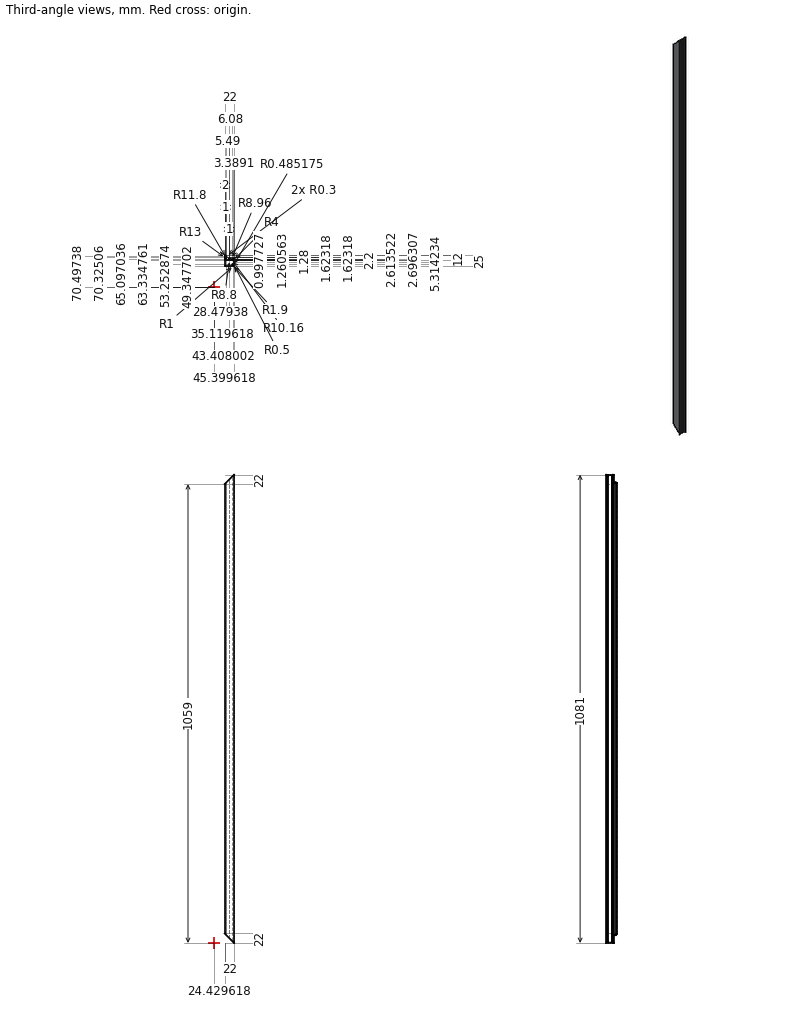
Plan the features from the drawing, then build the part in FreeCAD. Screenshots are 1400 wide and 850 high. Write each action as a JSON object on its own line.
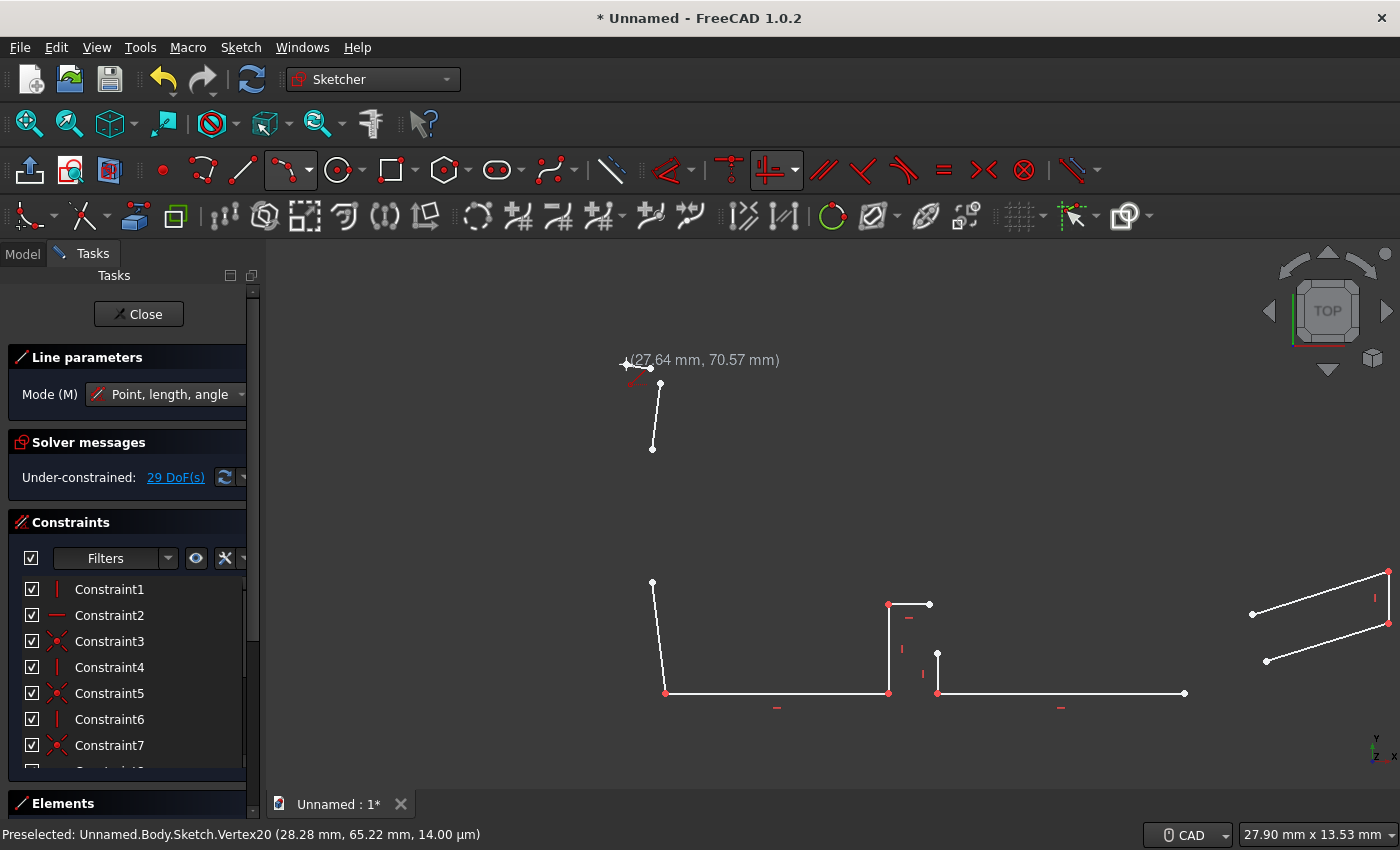
{"action": "left_click", "coordinate": [612, 375]}
{"action": "left_click", "coordinate": [603, 441]}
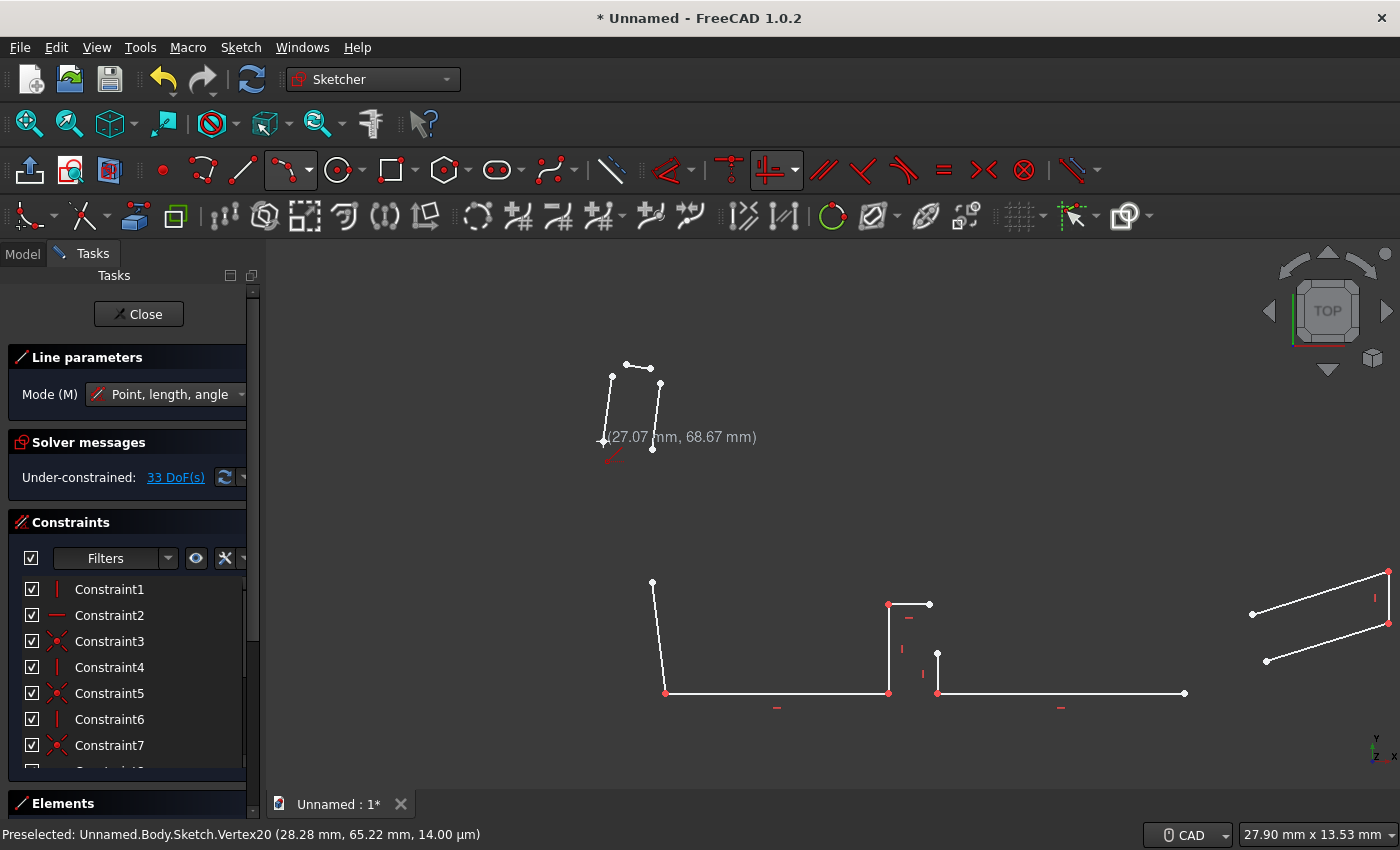
{"action": "left_click", "coordinate": [204, 170]}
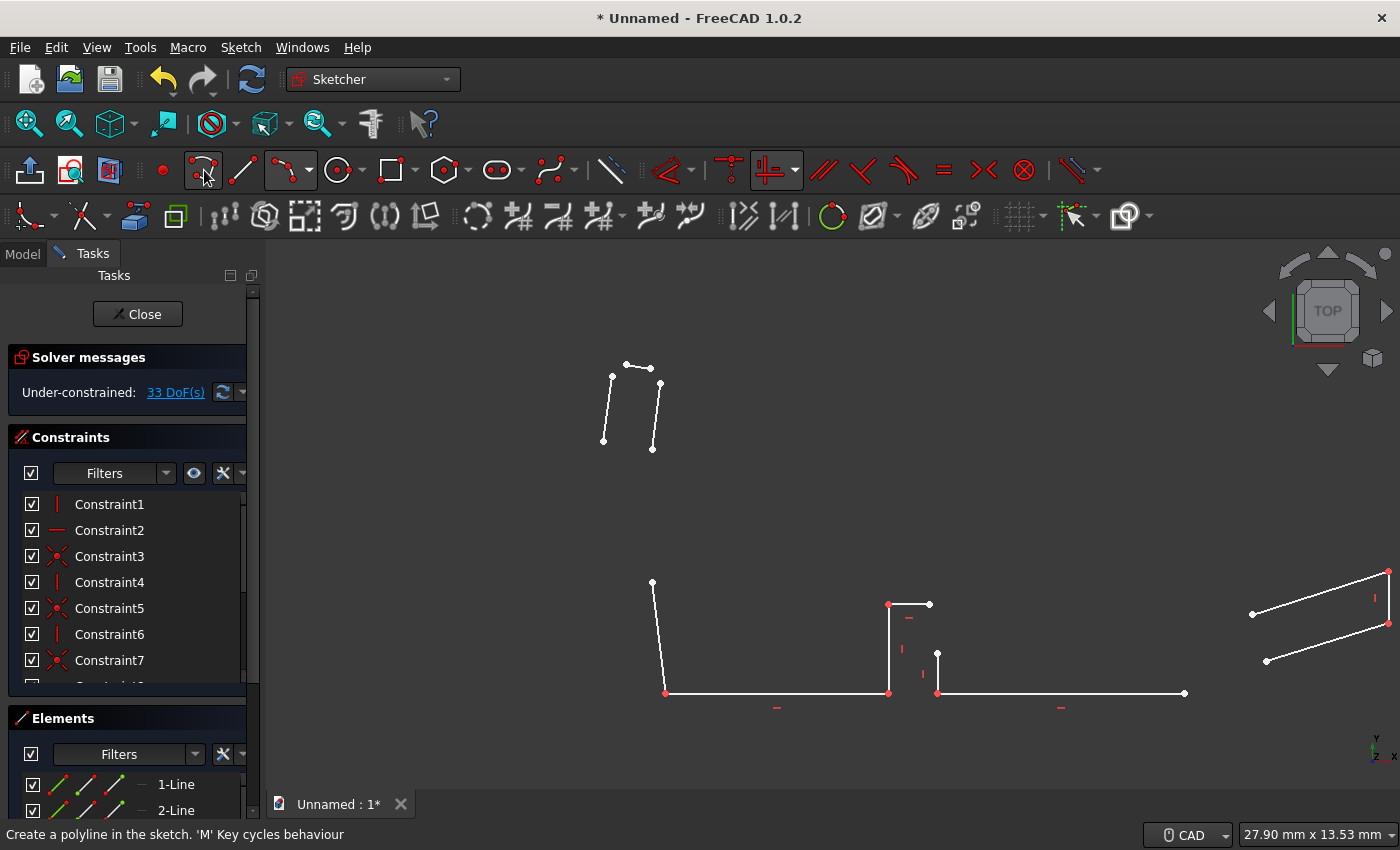
{"action": "left_click", "coordinate": [603, 587]}
{"action": "left_click", "coordinate": [618, 693]}
{"action": "left_click", "coordinate": [618, 745]}
{"action": "left_click", "coordinate": [577, 745]}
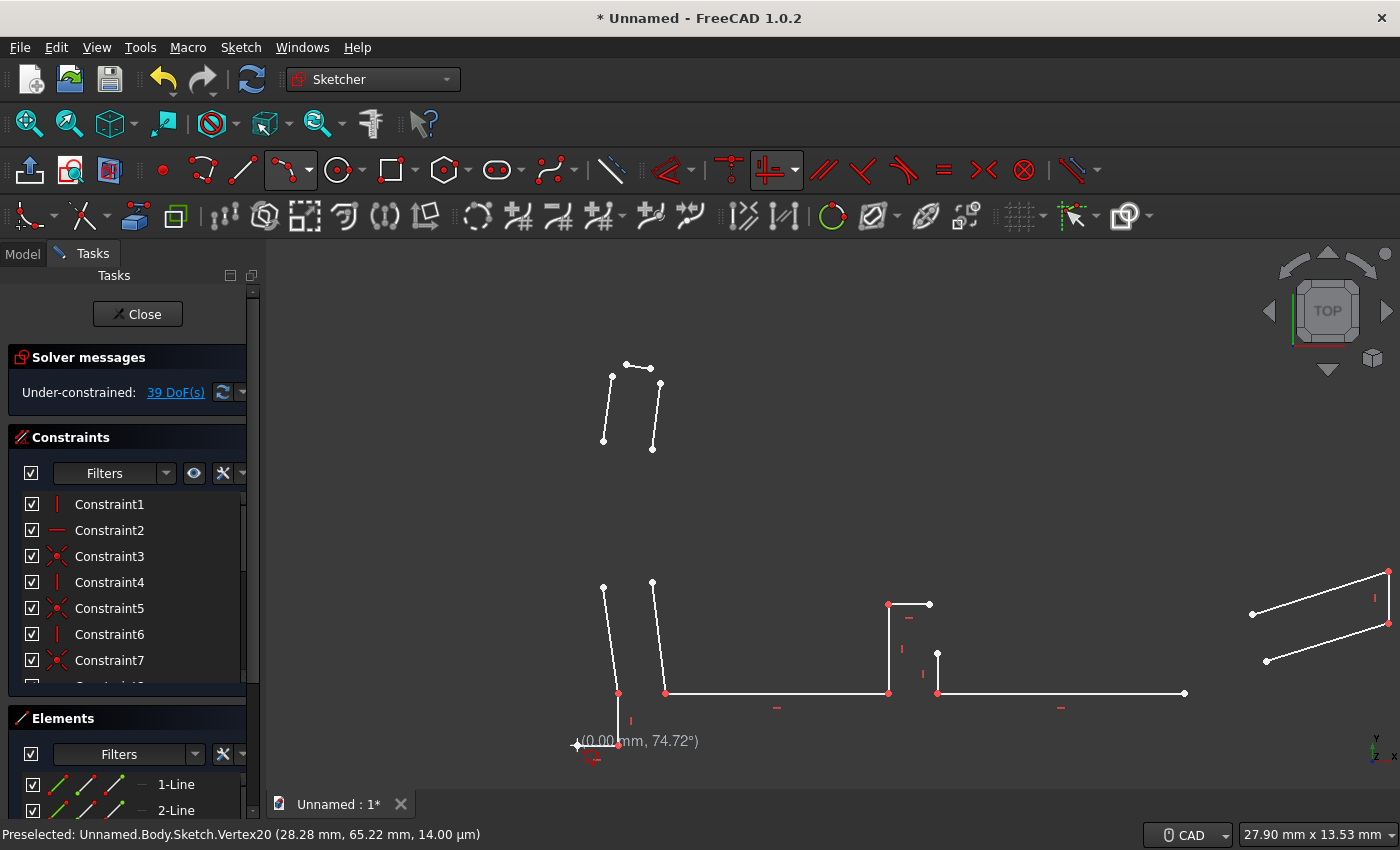
{"action": "scroll", "coordinate": [661, 367], "scroll_direction": "down", "scroll_amount": 5}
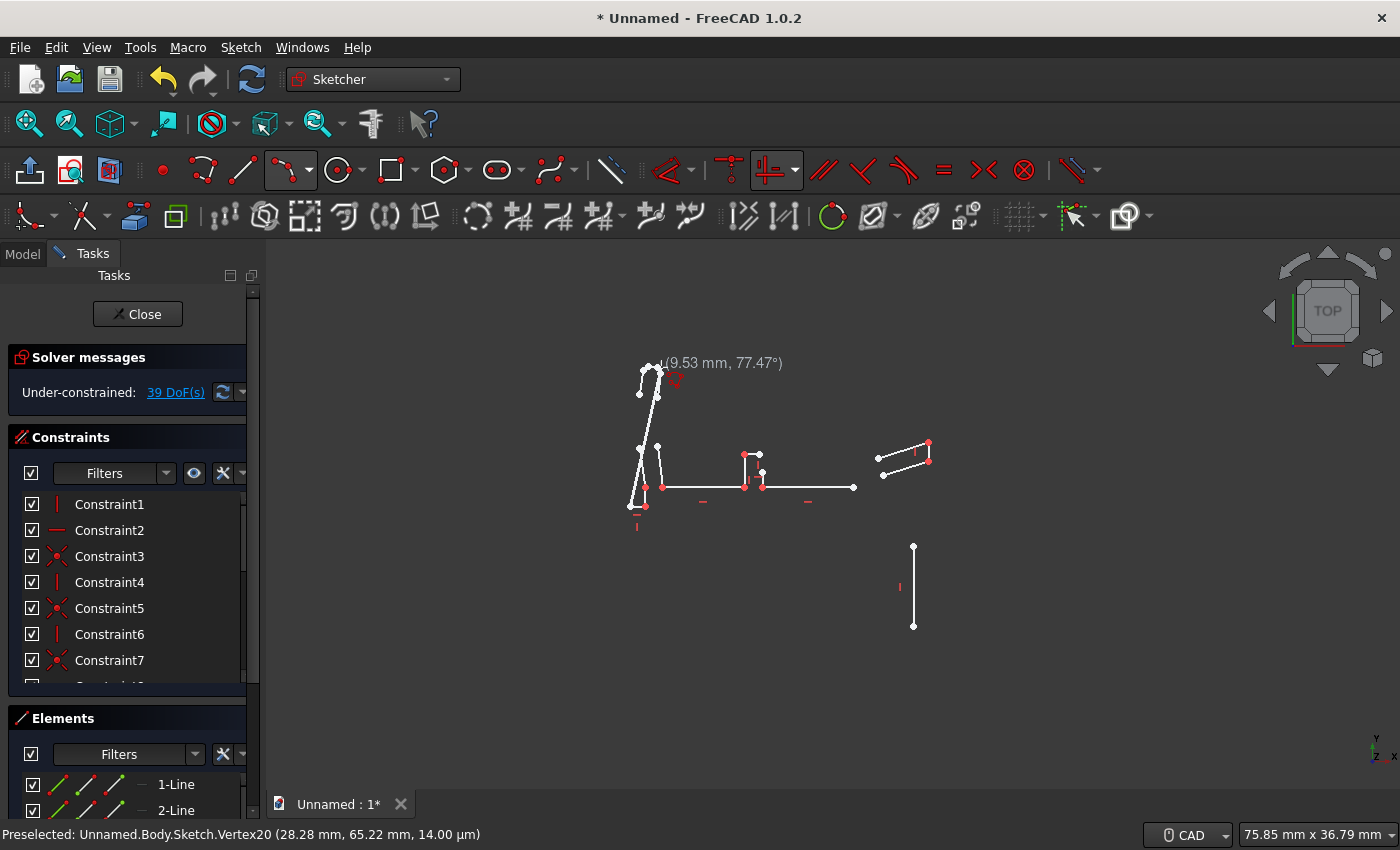
{"action": "left_click", "coordinate": [630, 327]}
{"action": "left_click", "coordinate": [600, 327]}
{"action": "left_click", "coordinate": [600, 701]}
{"action": "left_click", "coordinate": [929, 701]}
{"action": "right_click", "coordinate": [929, 701]}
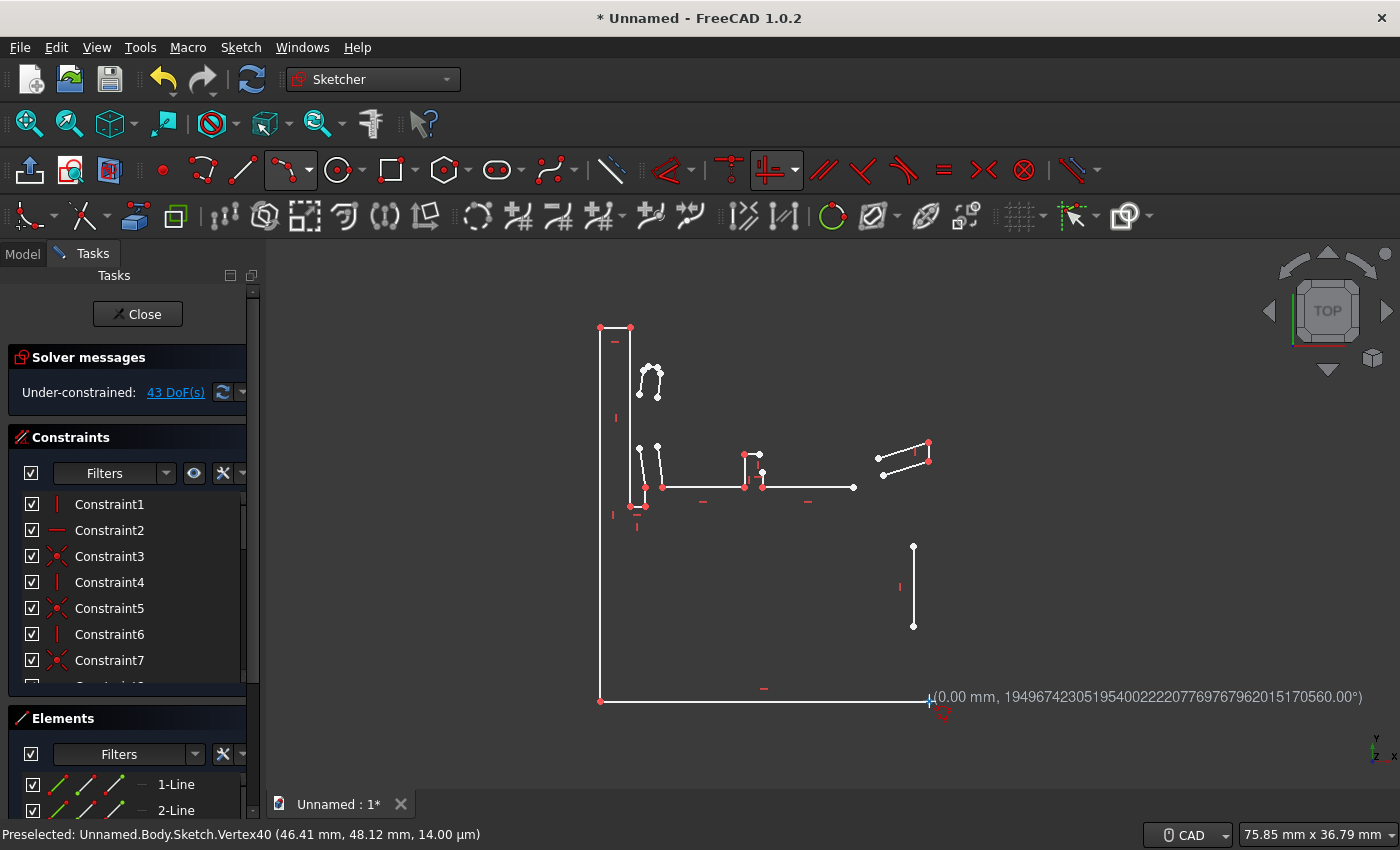
{"action": "key", "text": "g 3 a"}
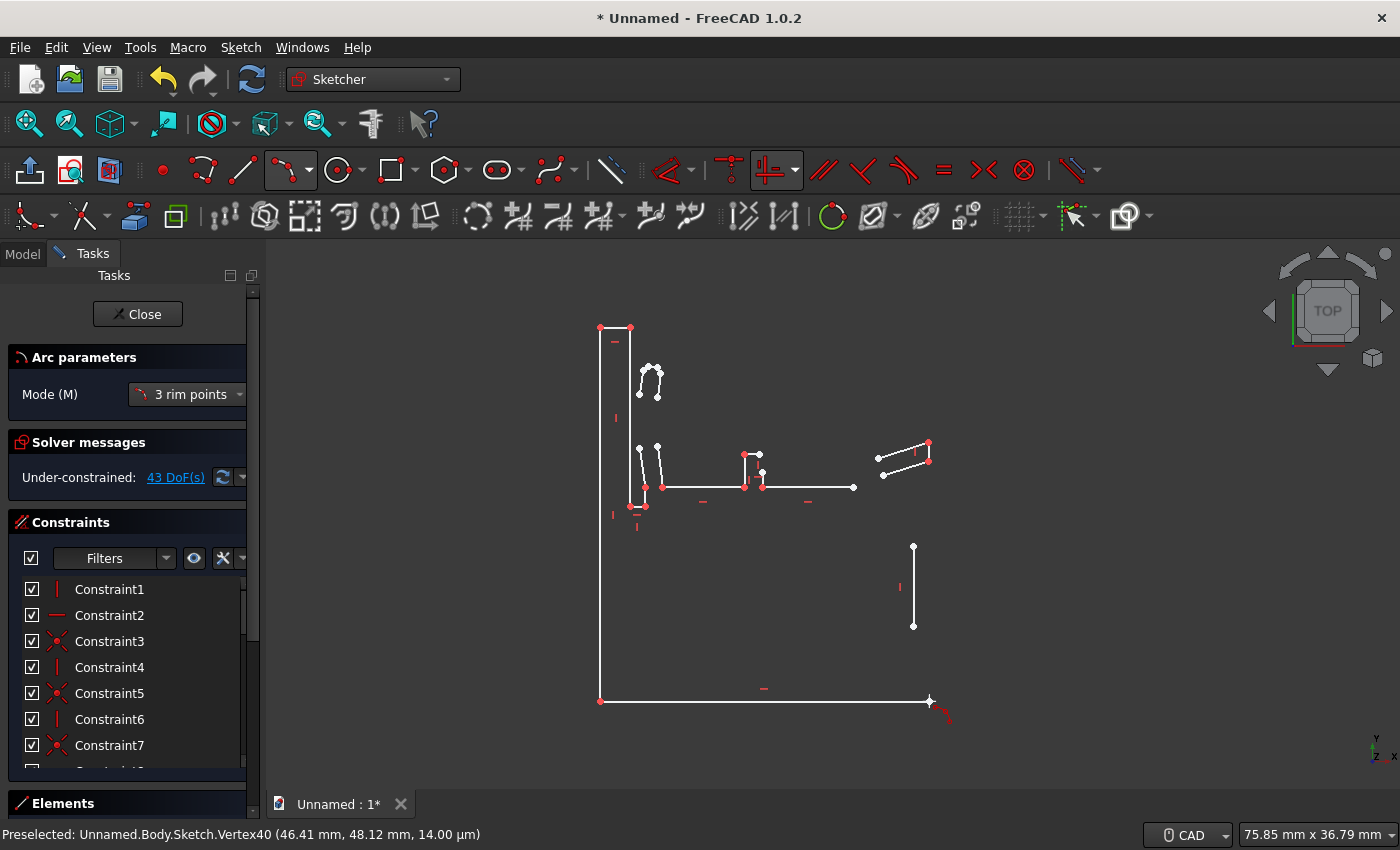
{"action": "left_click", "coordinate": [914, 546]}
{"action": "left_click", "coordinate": [854, 487]}
{"action": "left_click", "coordinate": [896, 504]}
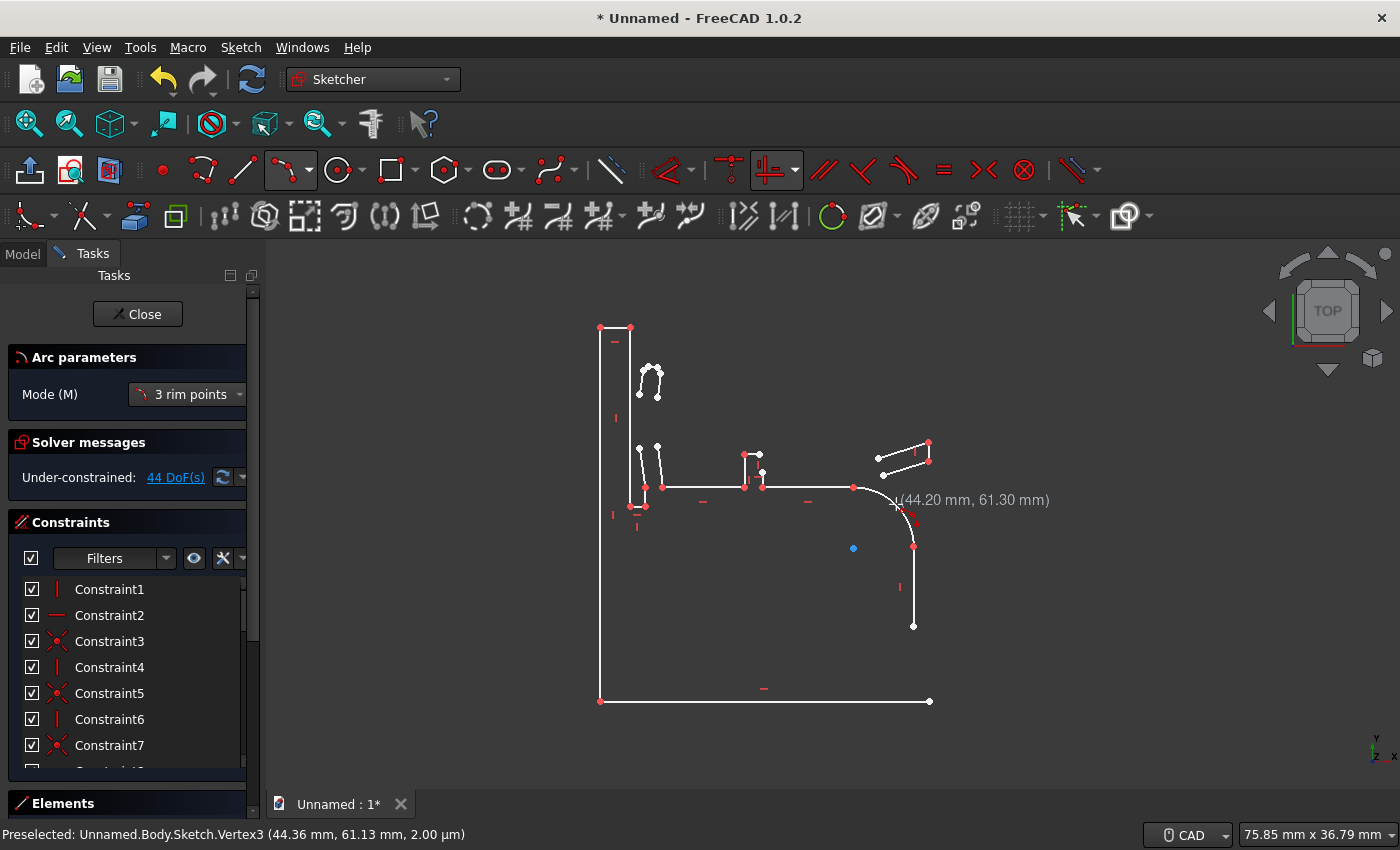
{"action": "scroll", "coordinate": [763, 471], "scroll_direction": "up", "scroll_amount": 4}